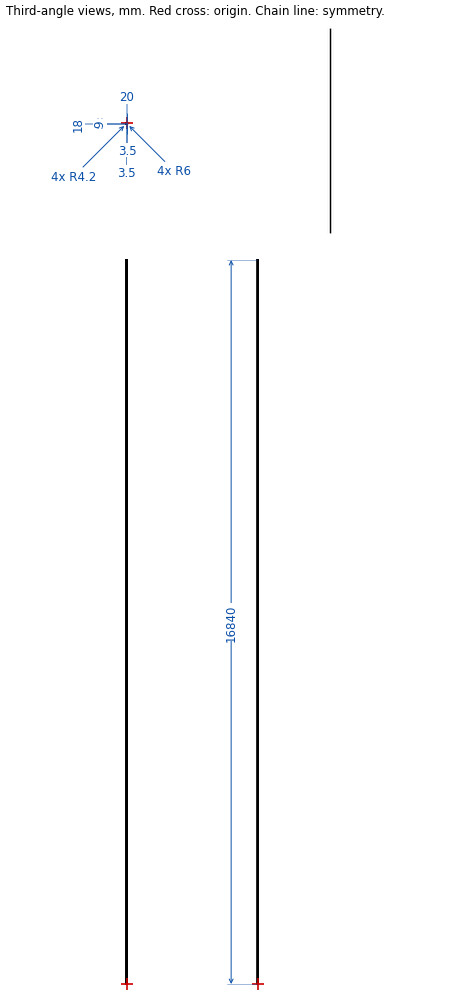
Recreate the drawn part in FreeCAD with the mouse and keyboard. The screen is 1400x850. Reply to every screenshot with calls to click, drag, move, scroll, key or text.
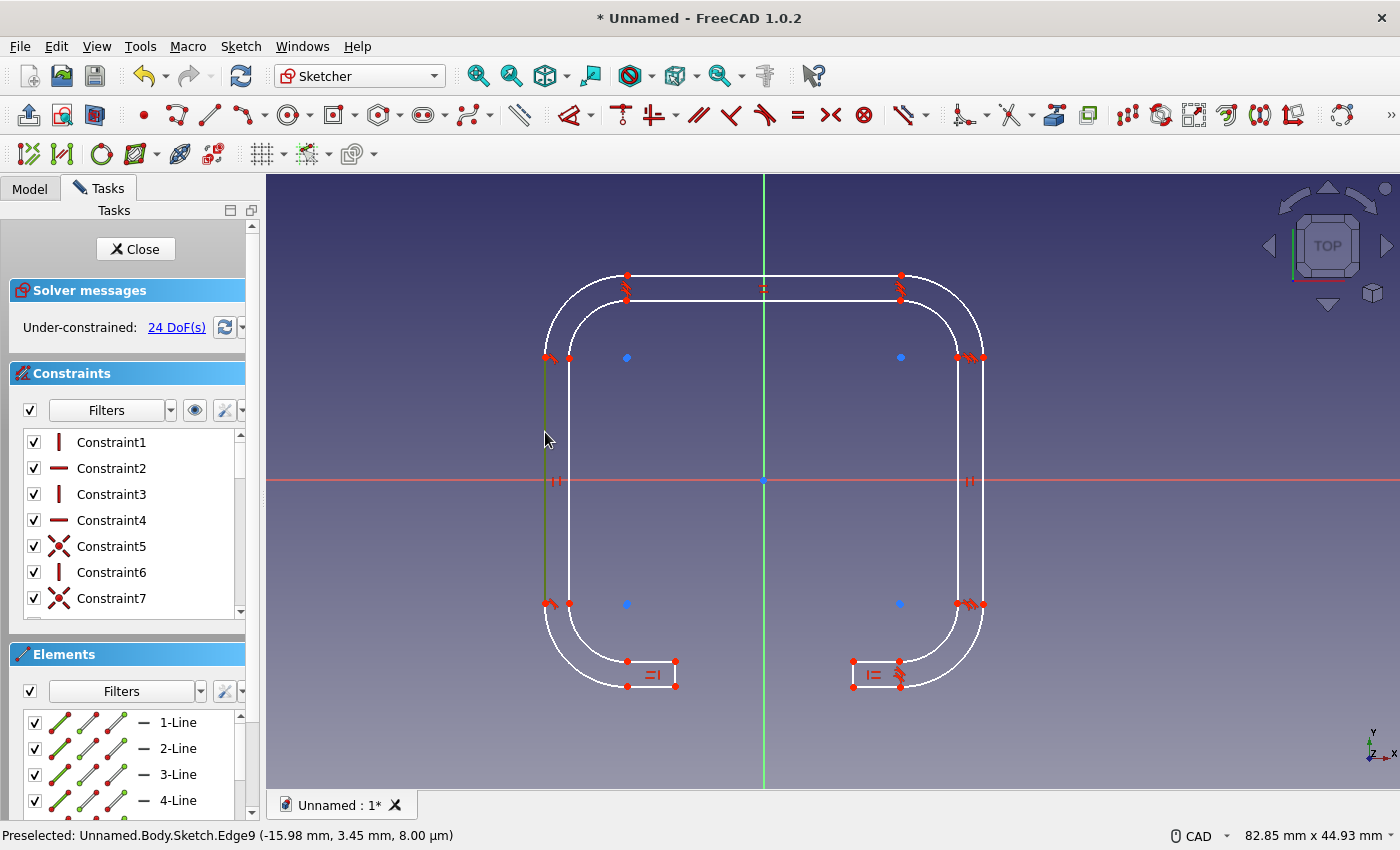
click(590, 285)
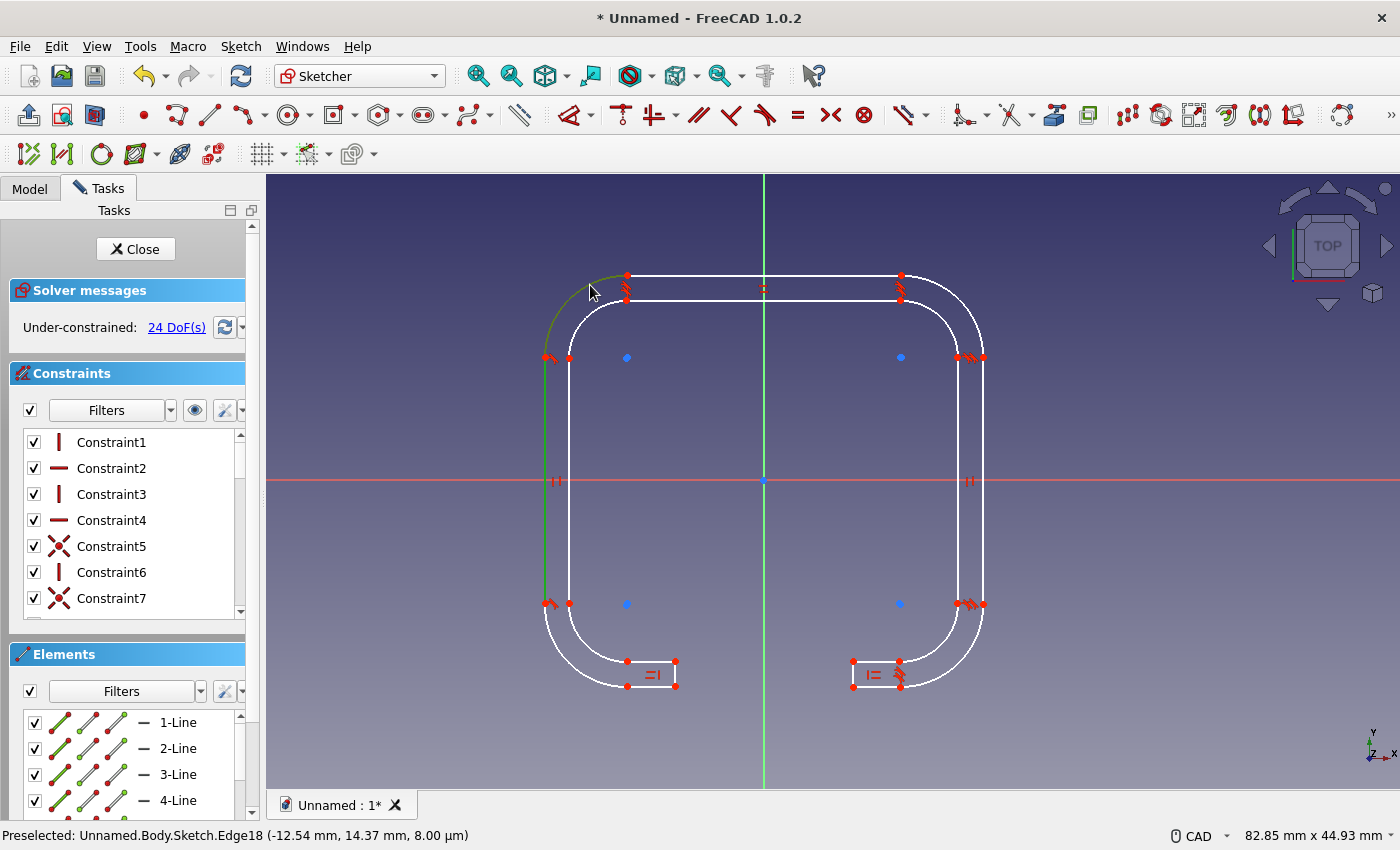
click(765, 116)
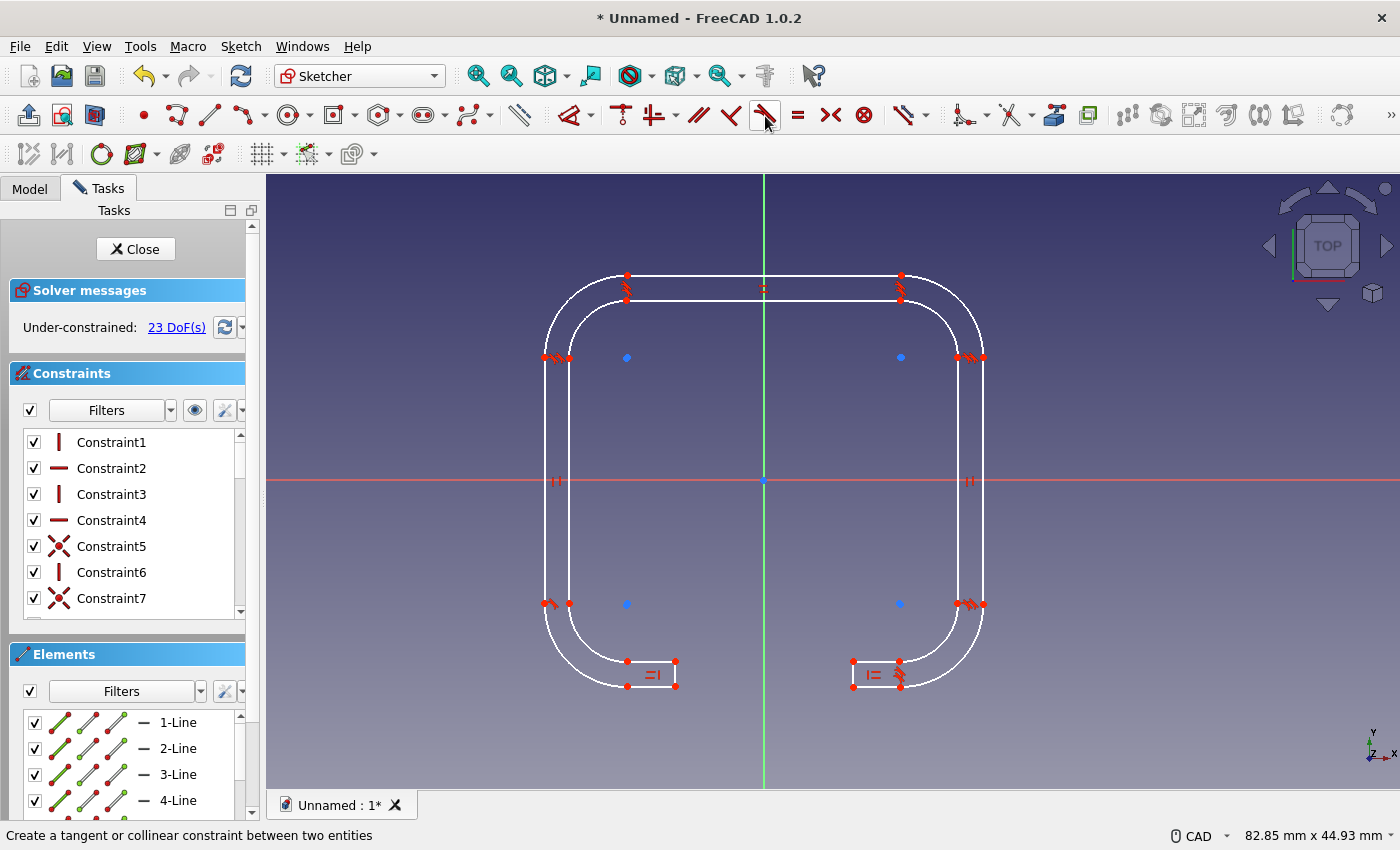
click(545, 432)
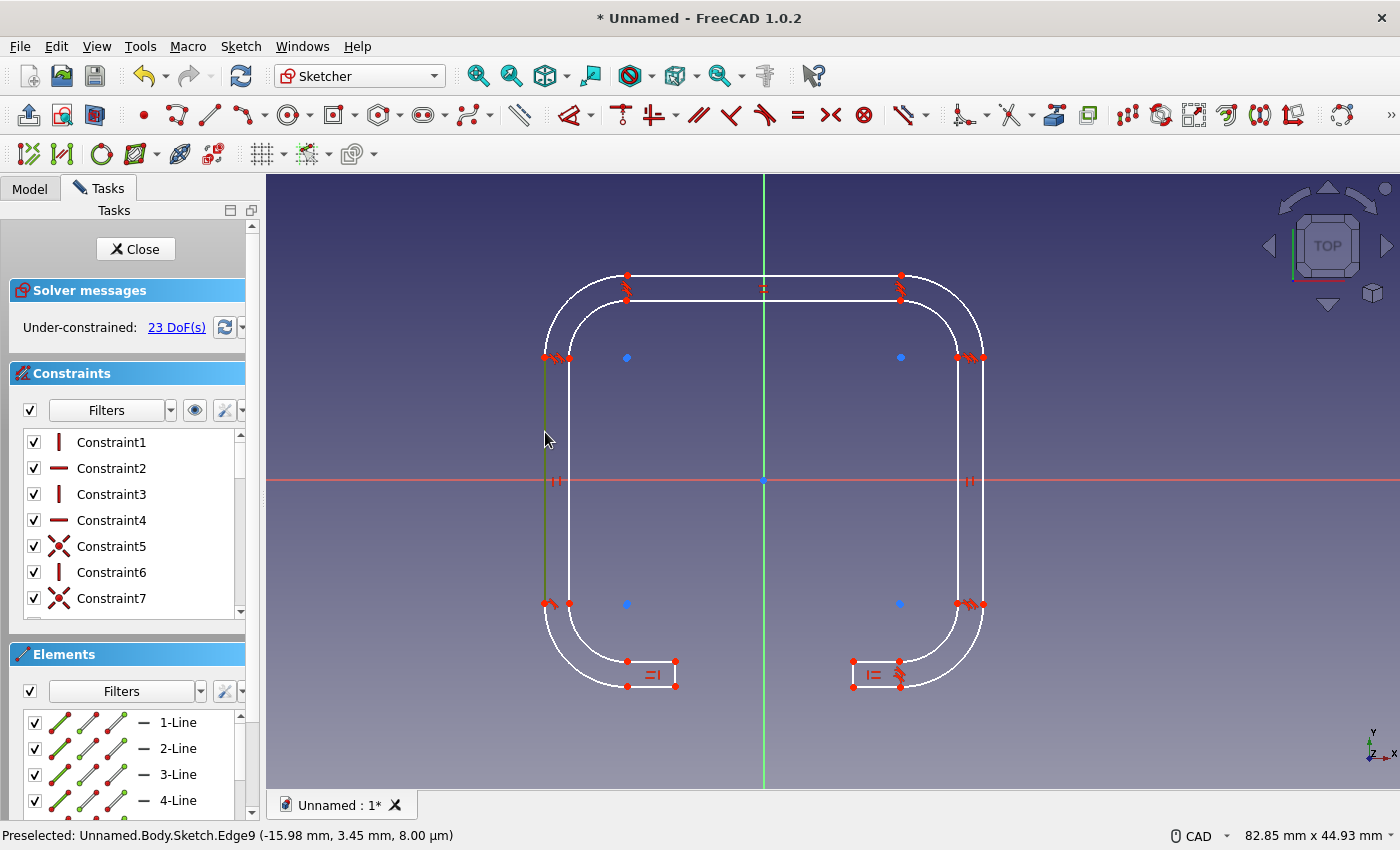
click(554, 642)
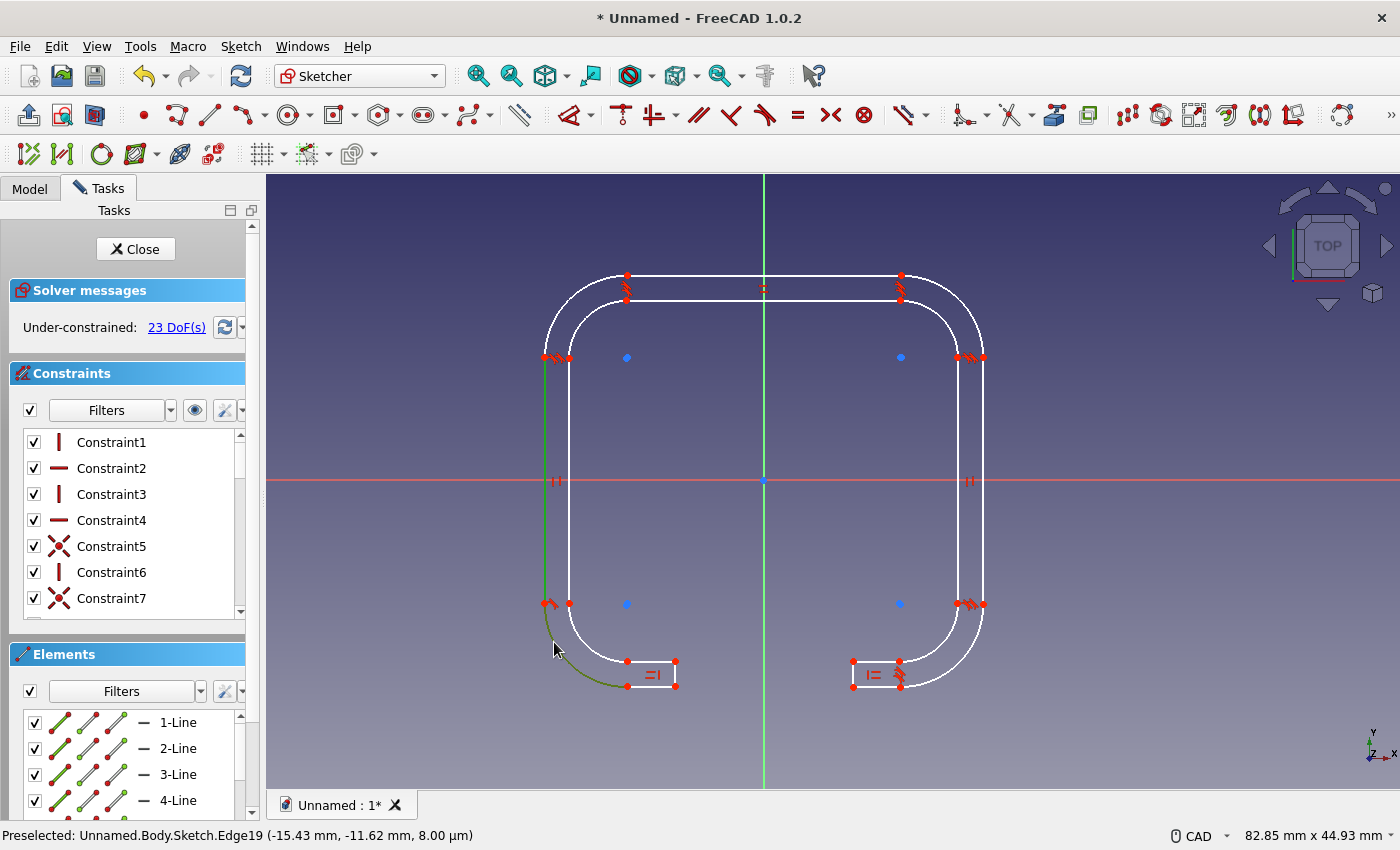
click(765, 116)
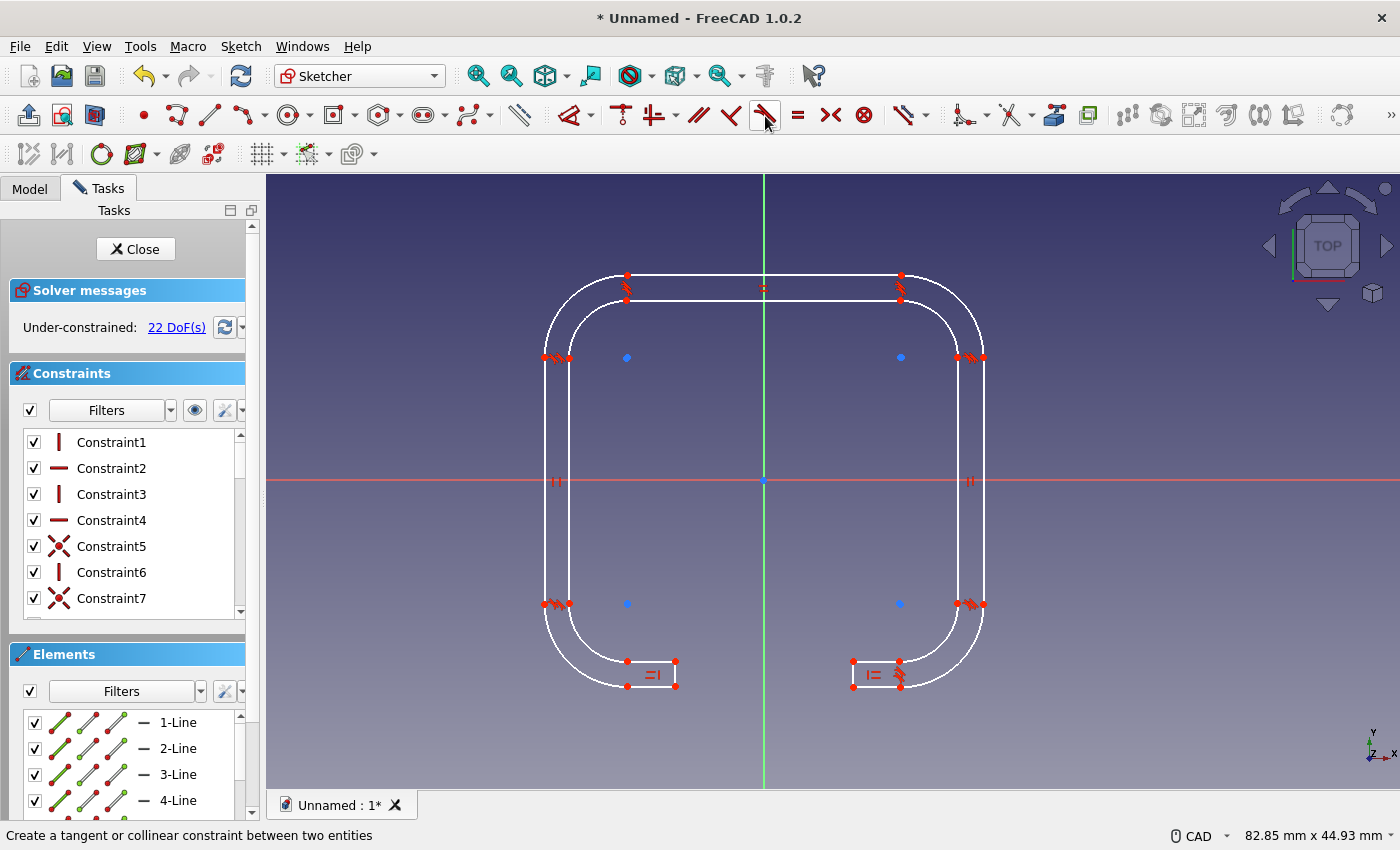
click(641, 687)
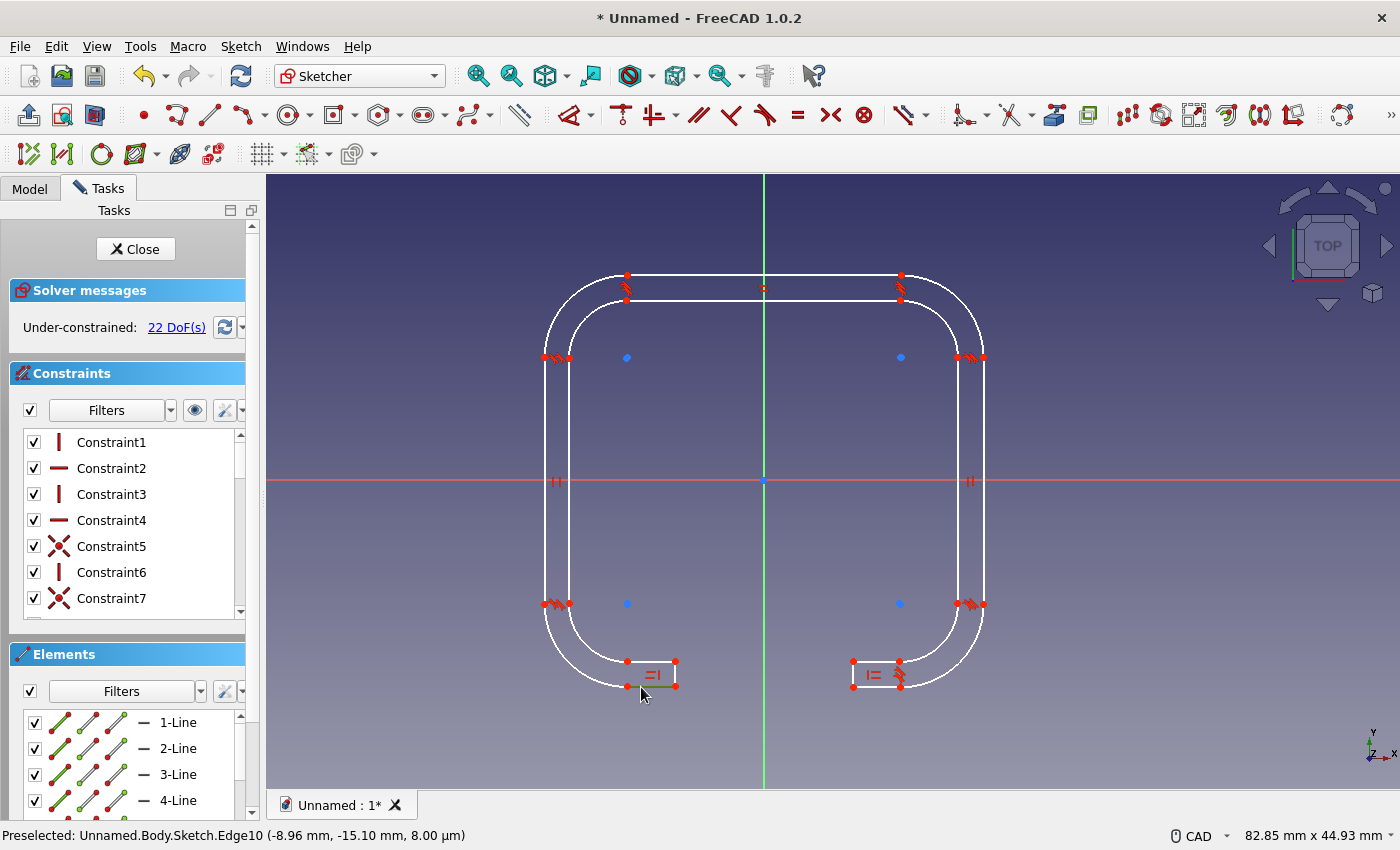
click(554, 641)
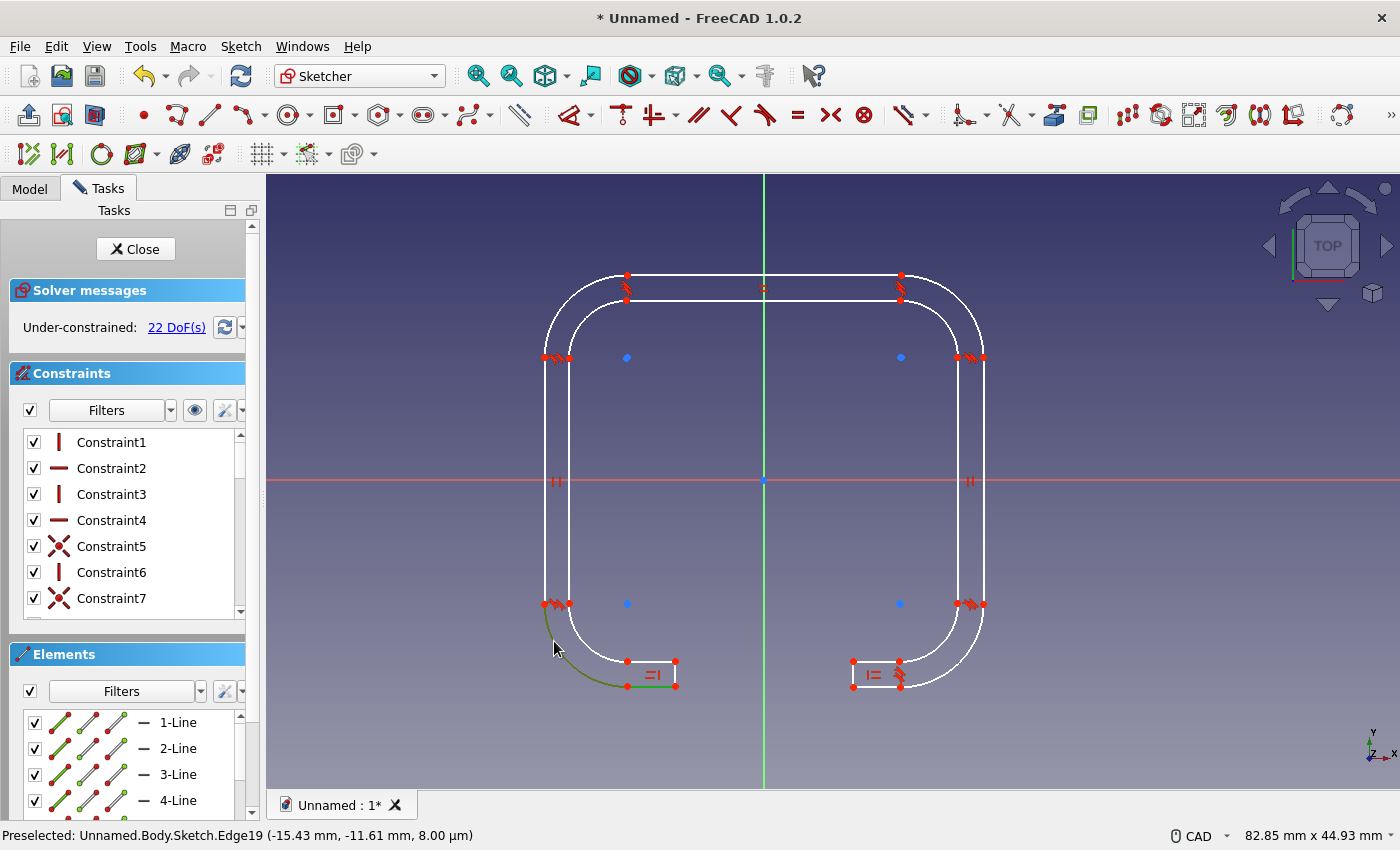
click(765, 116)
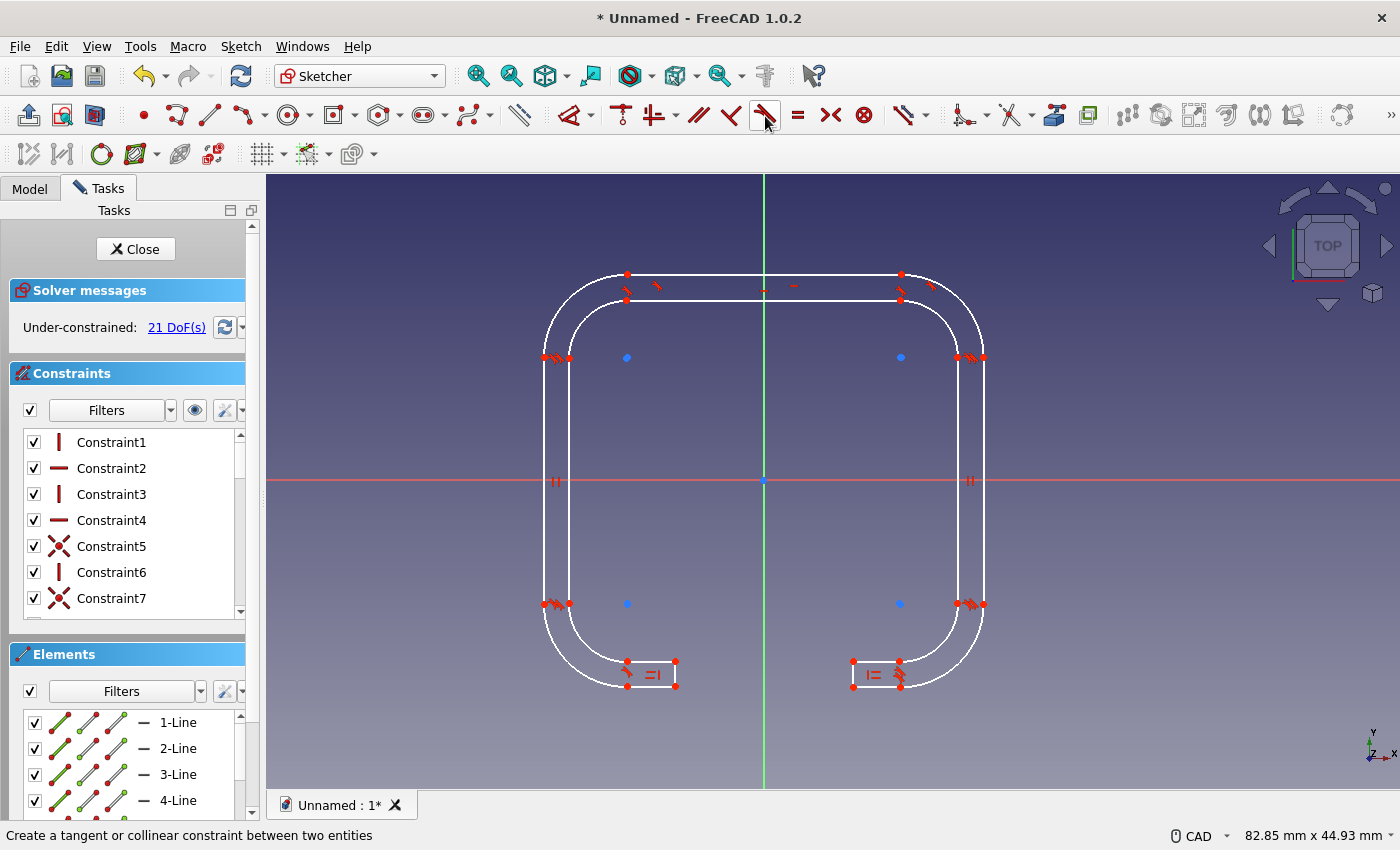
click(661, 662)